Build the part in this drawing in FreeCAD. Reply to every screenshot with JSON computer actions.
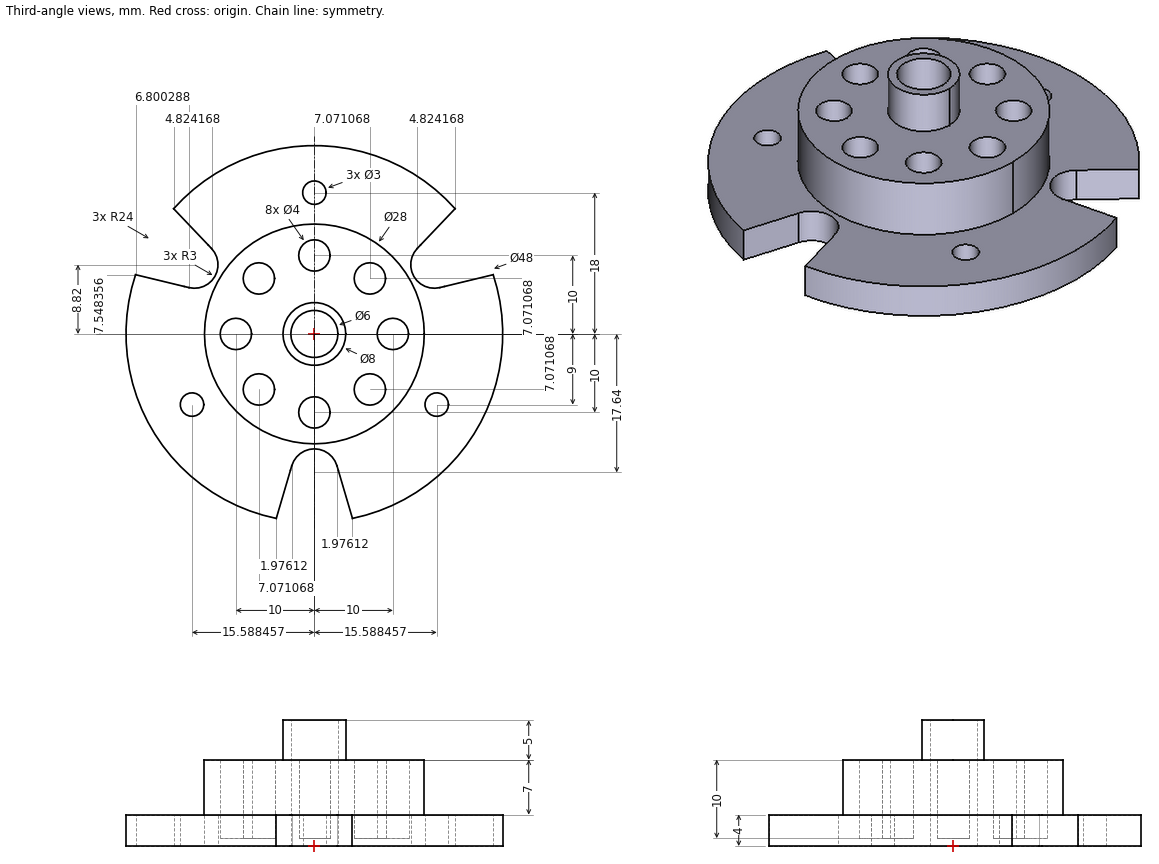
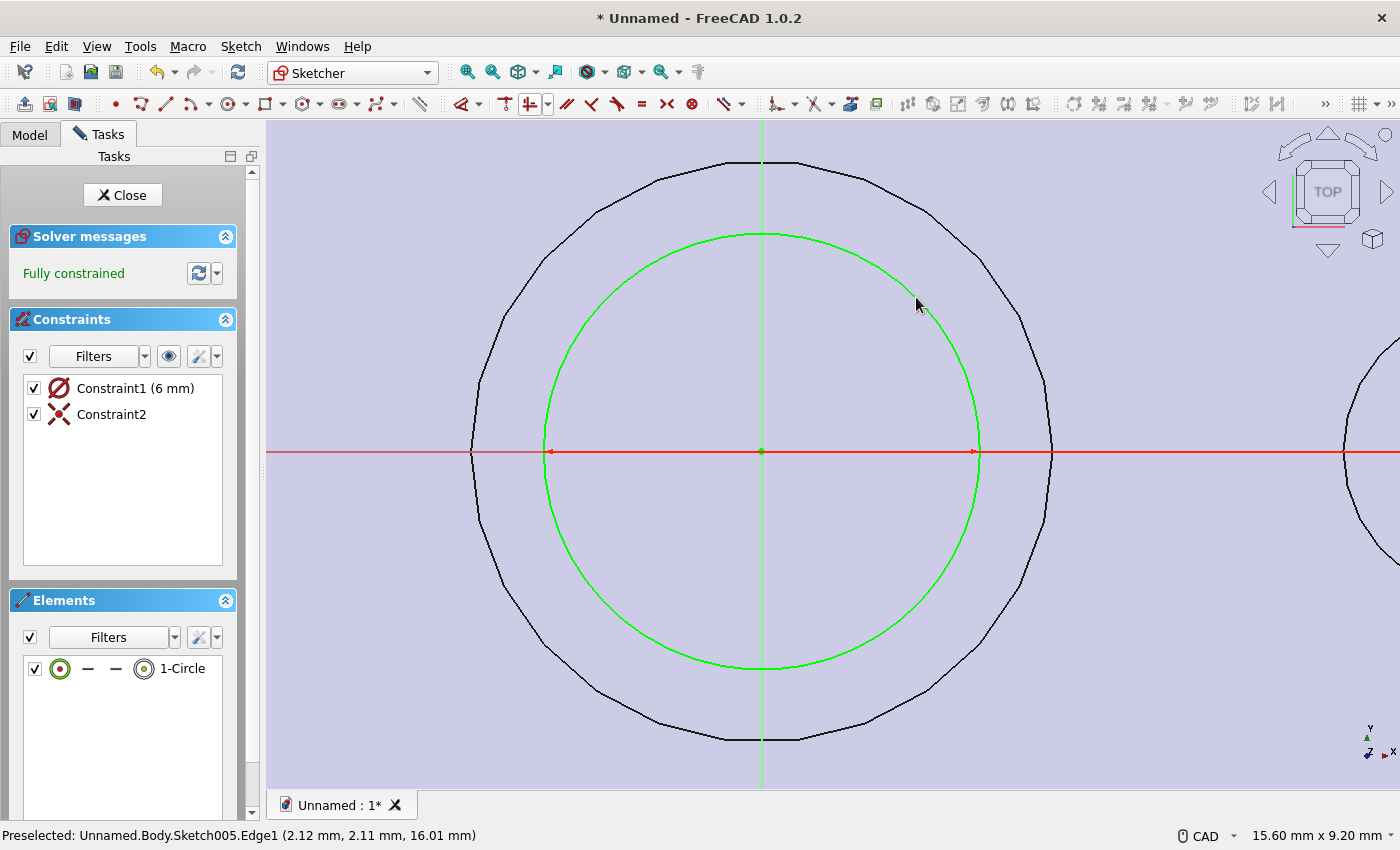
{"action": "left_click", "coordinate": [123, 195]}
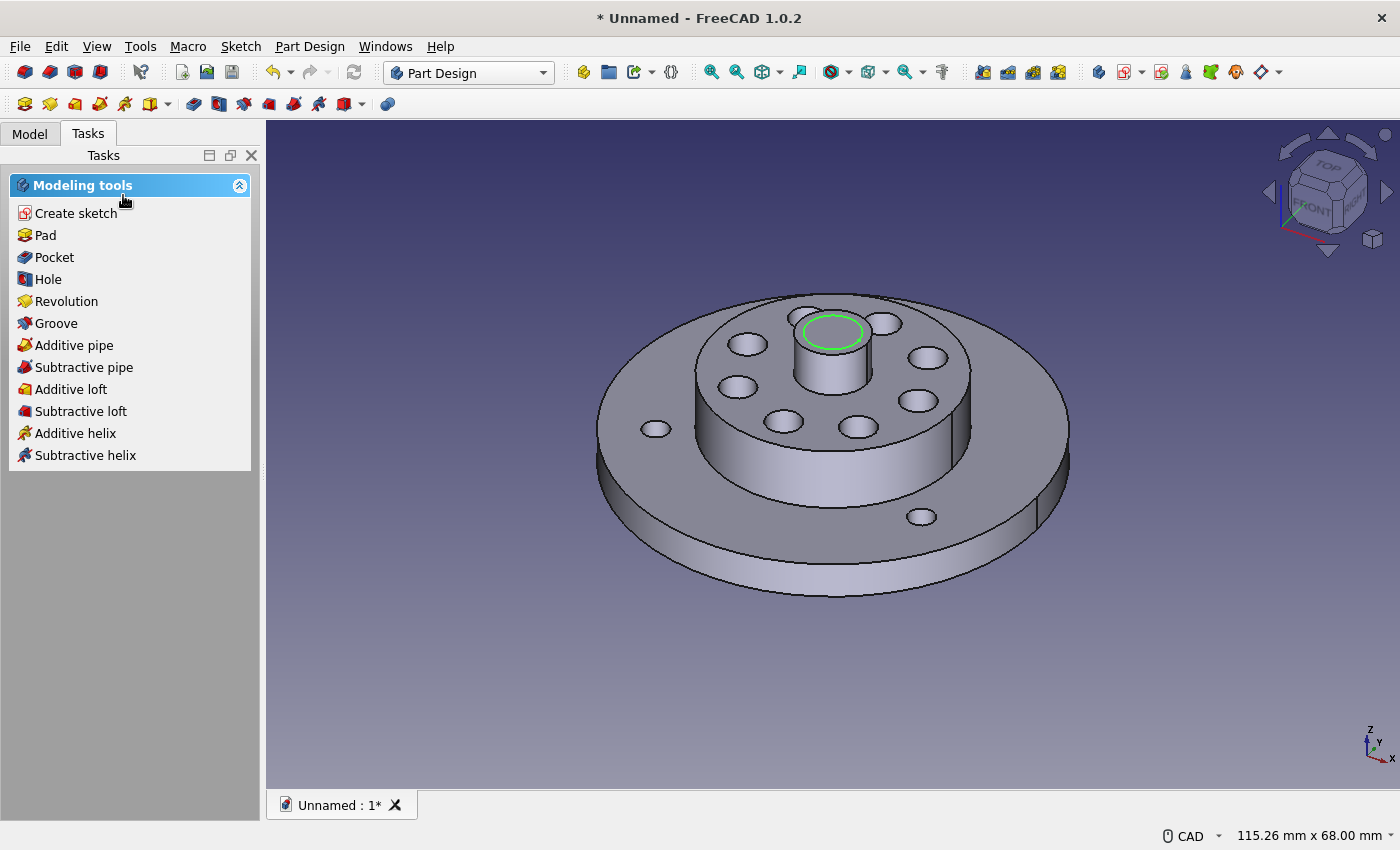
{"action": "left_click", "coordinate": [194, 104]}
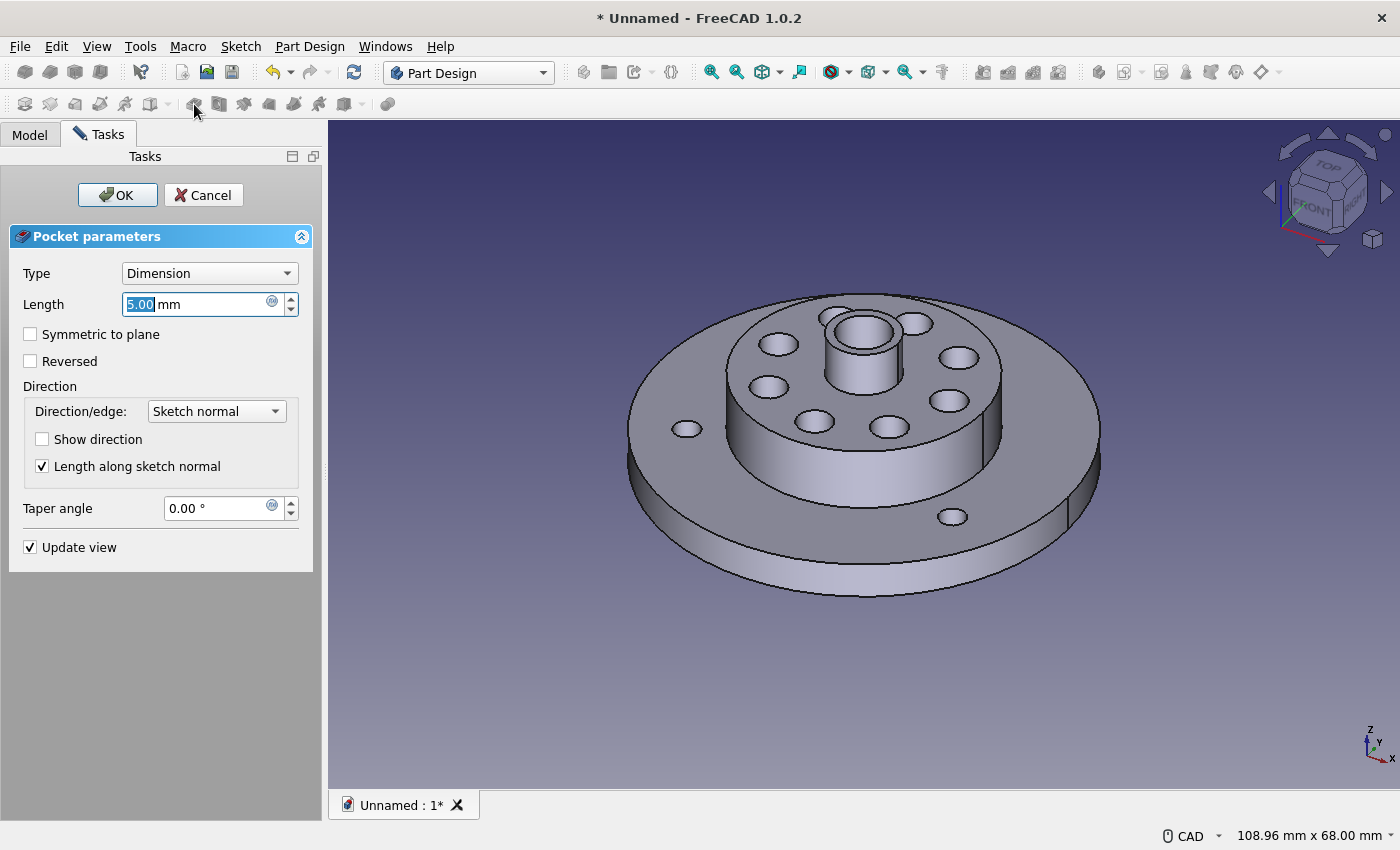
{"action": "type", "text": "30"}
{"action": "key", "text": "Tab"}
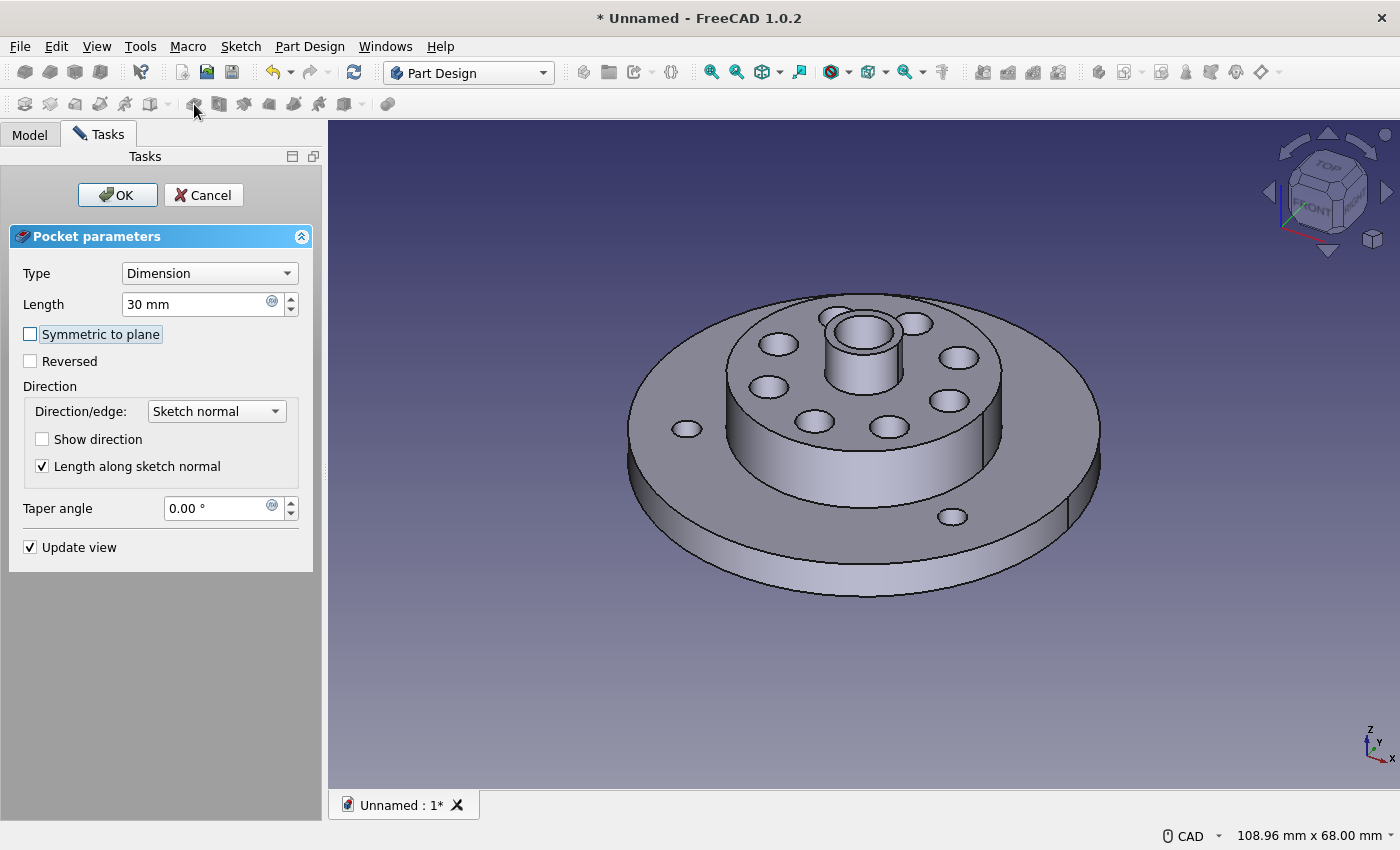
{"action": "left_click", "coordinate": [118, 195]}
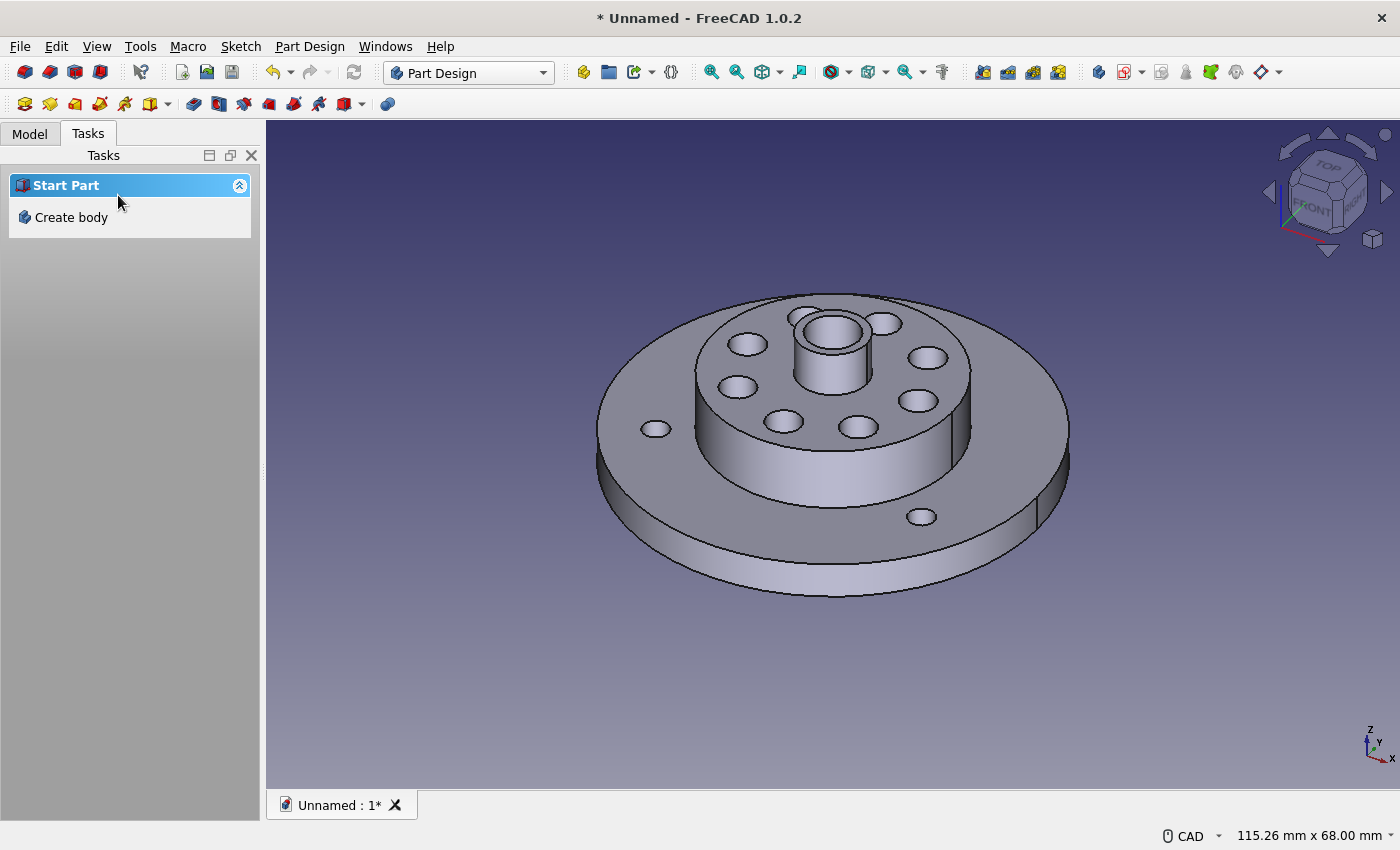
{"action": "left_click", "coordinate": [30, 134]}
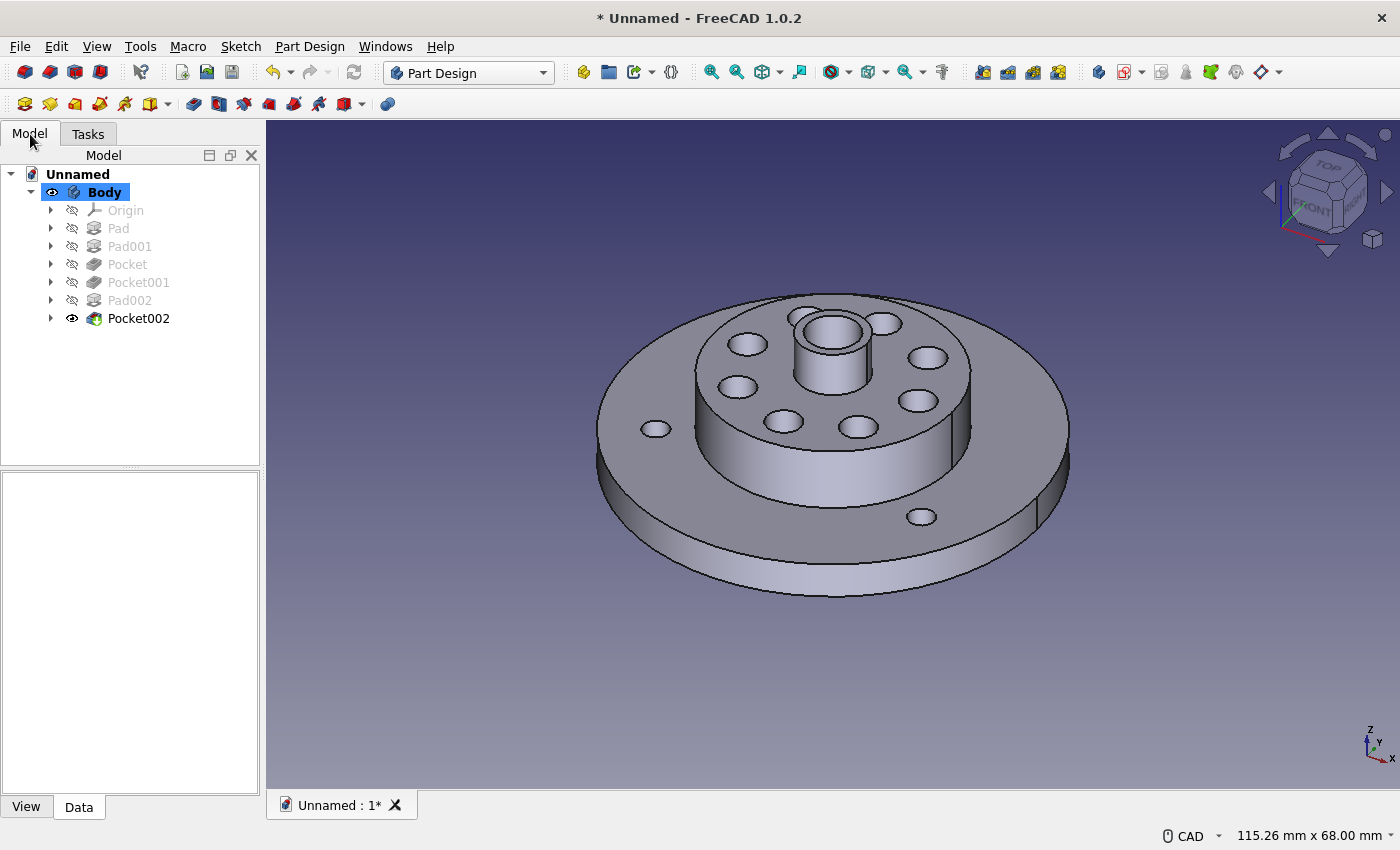
{"action": "left_click", "coordinate": [51, 210]}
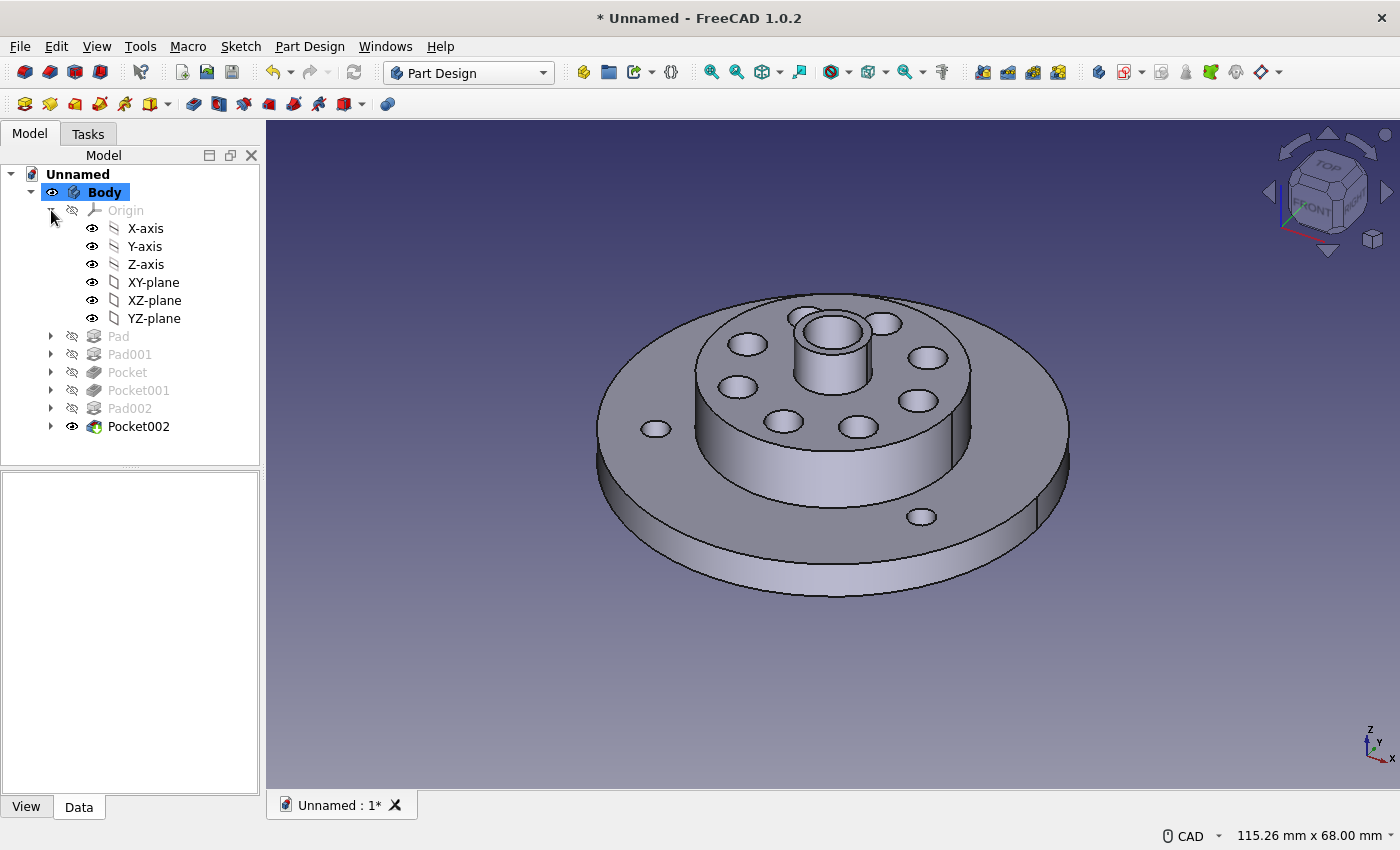
{"action": "left_click", "coordinate": [137, 282]}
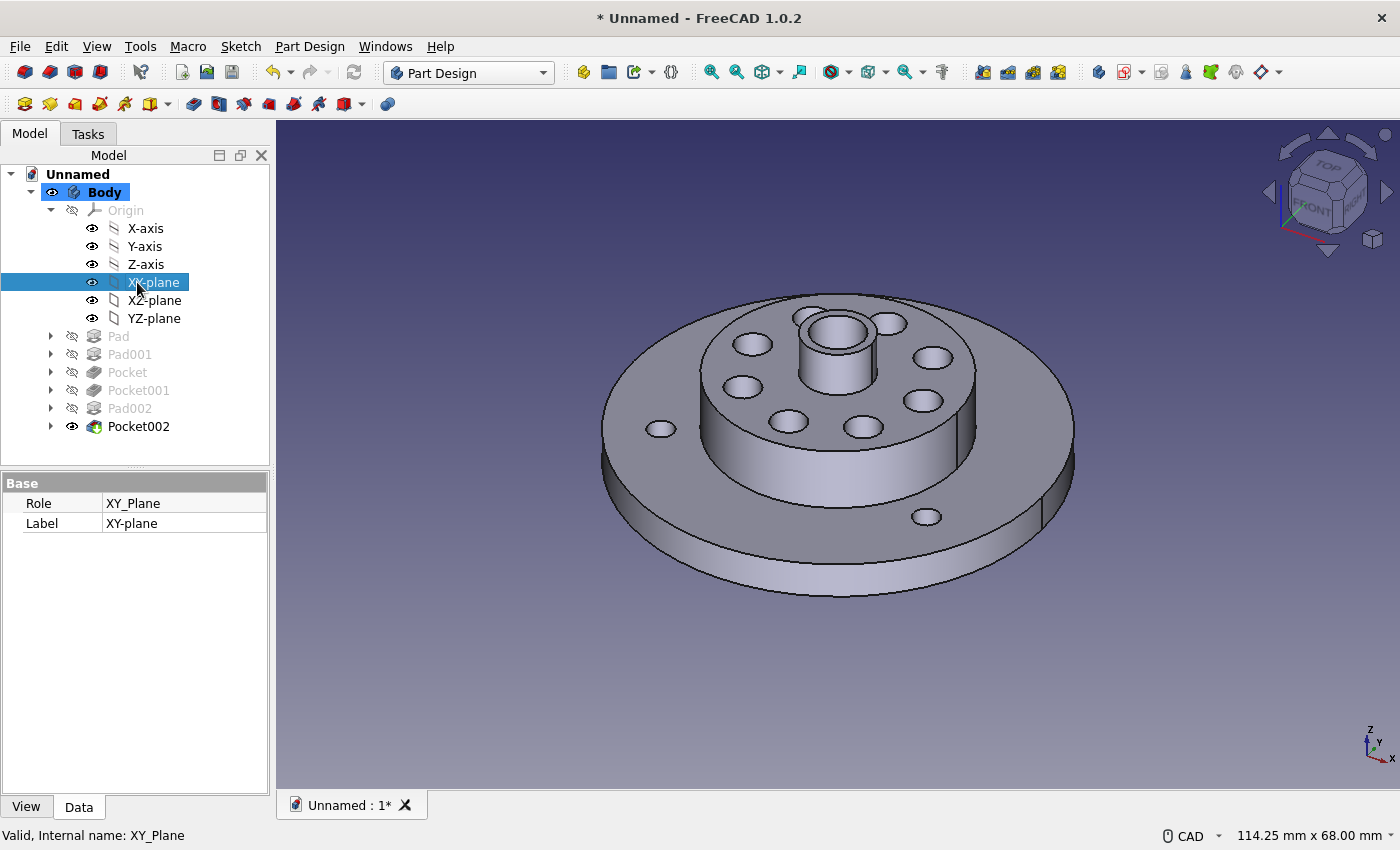
{"action": "left_click", "coordinate": [1260, 72]}